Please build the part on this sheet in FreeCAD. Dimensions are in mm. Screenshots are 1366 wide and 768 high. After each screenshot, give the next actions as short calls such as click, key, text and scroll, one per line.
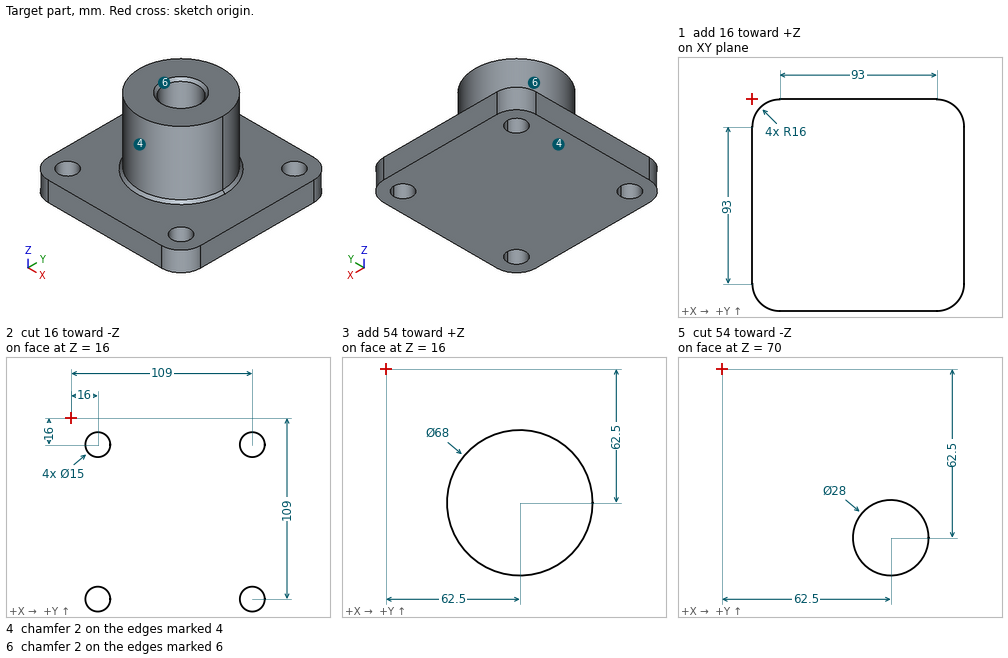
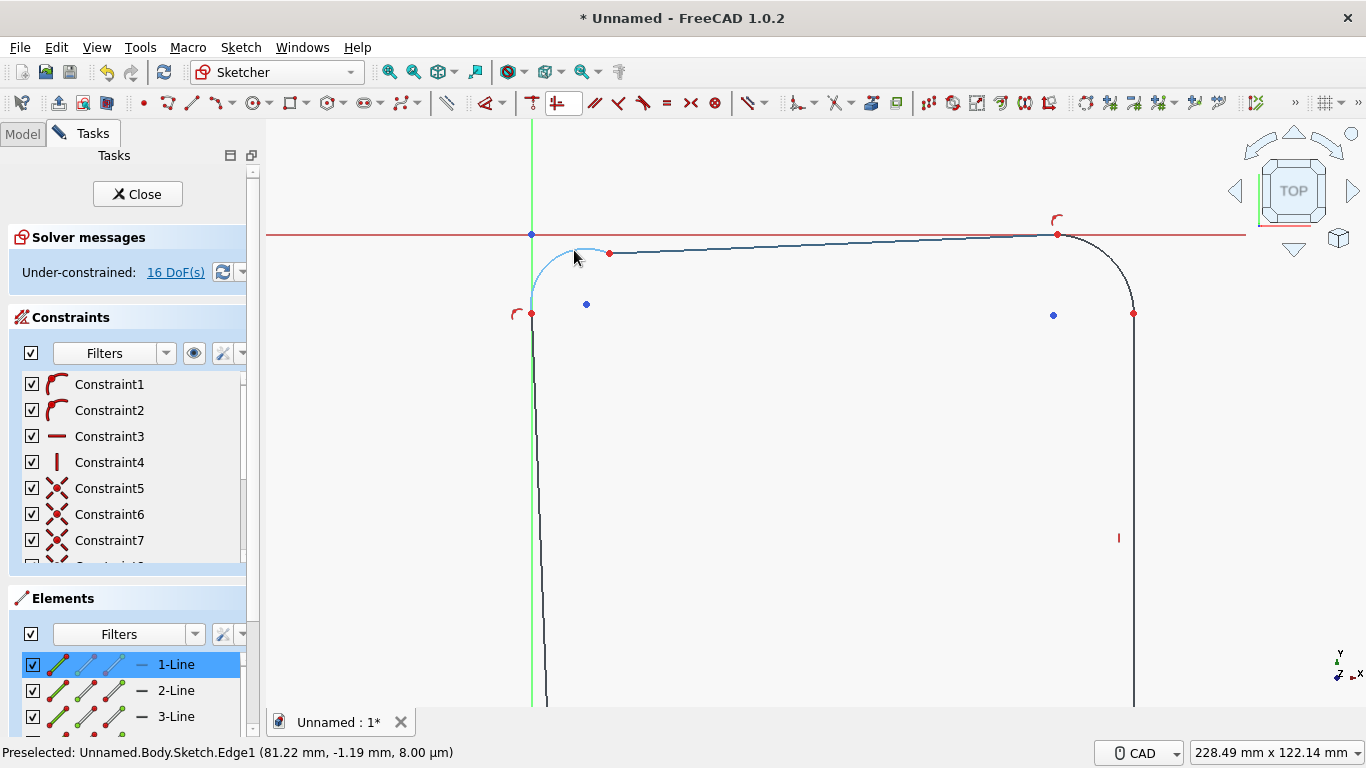
click(574, 250)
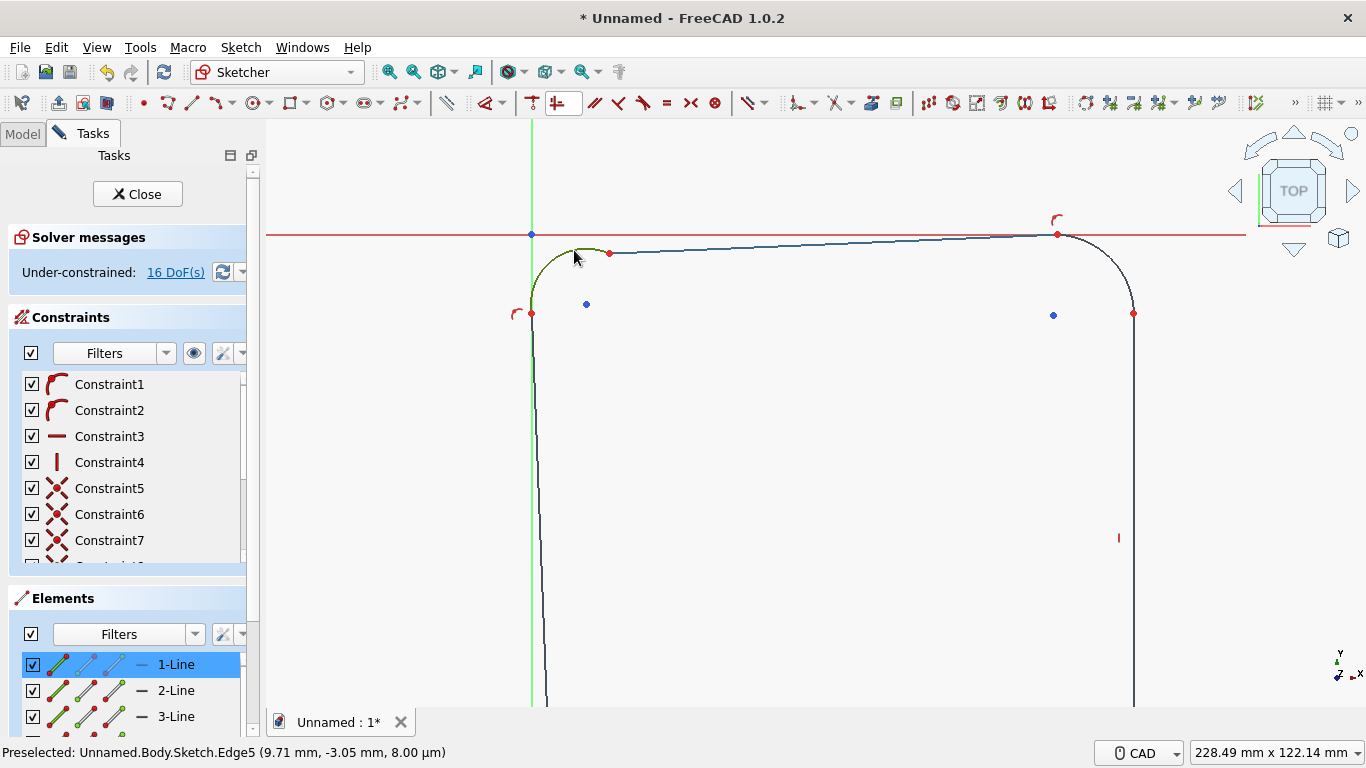
key(t)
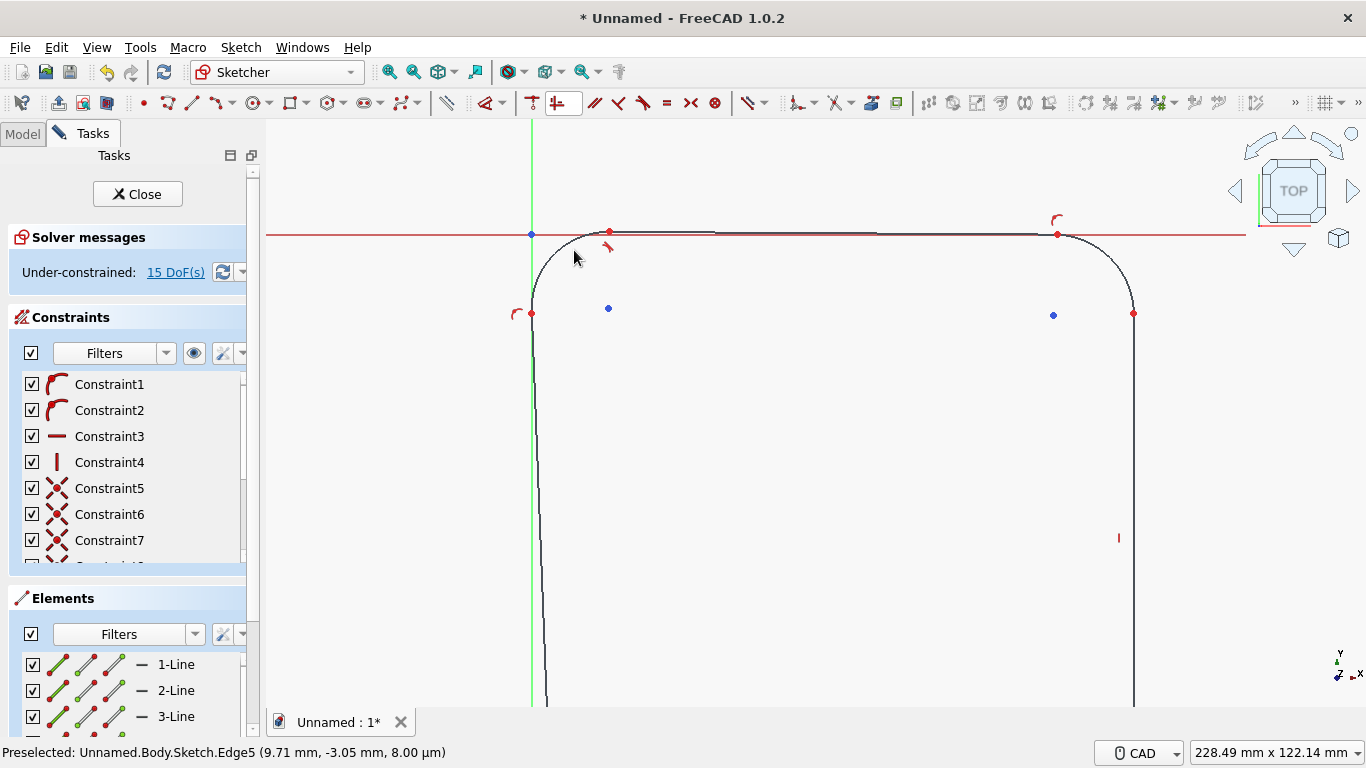
click(923, 234)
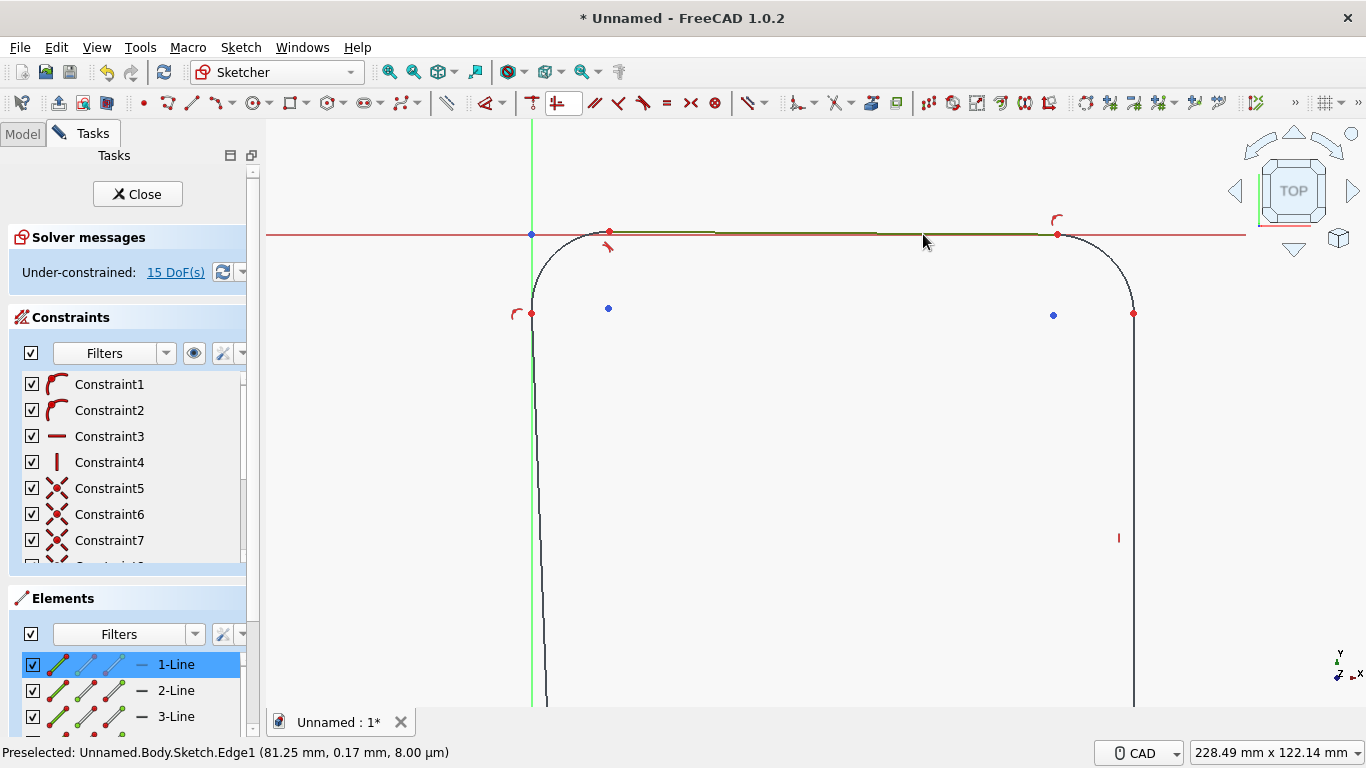
click(1125, 279)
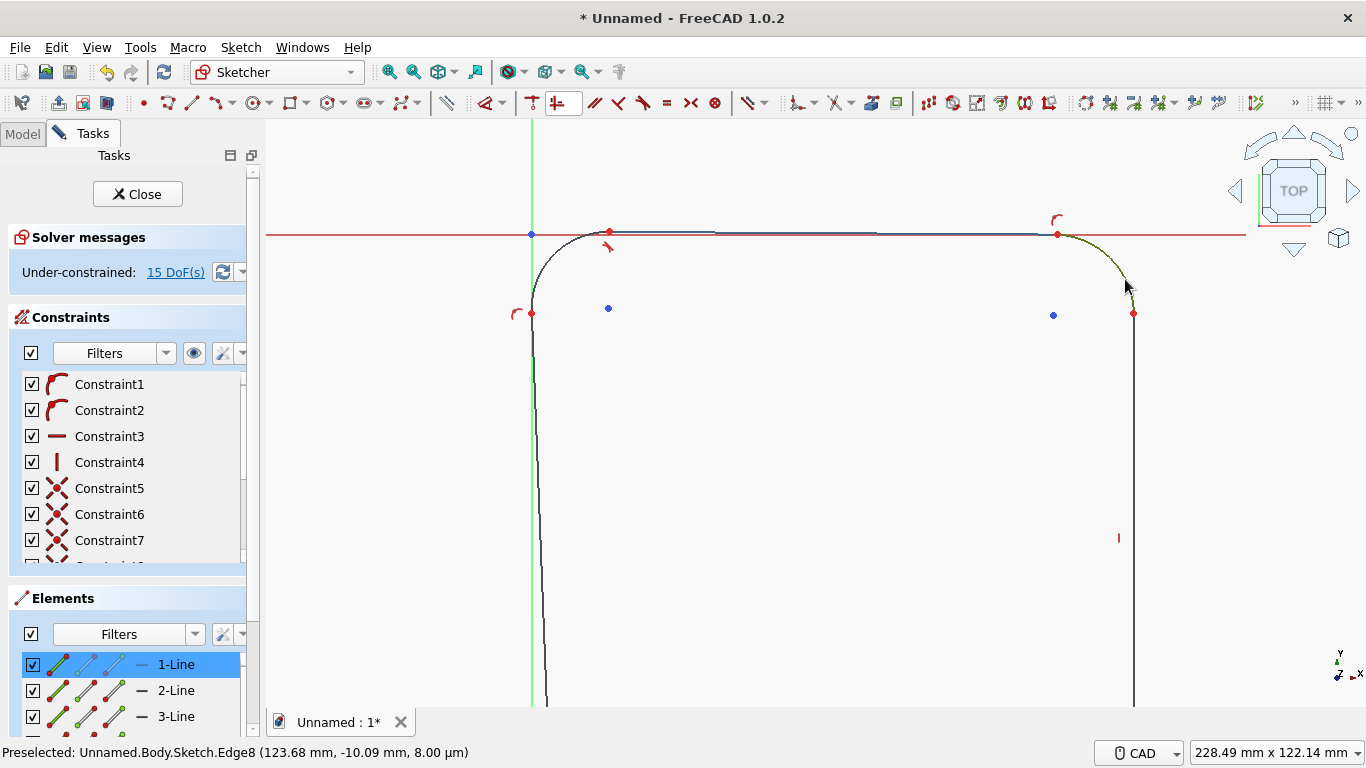
key(t)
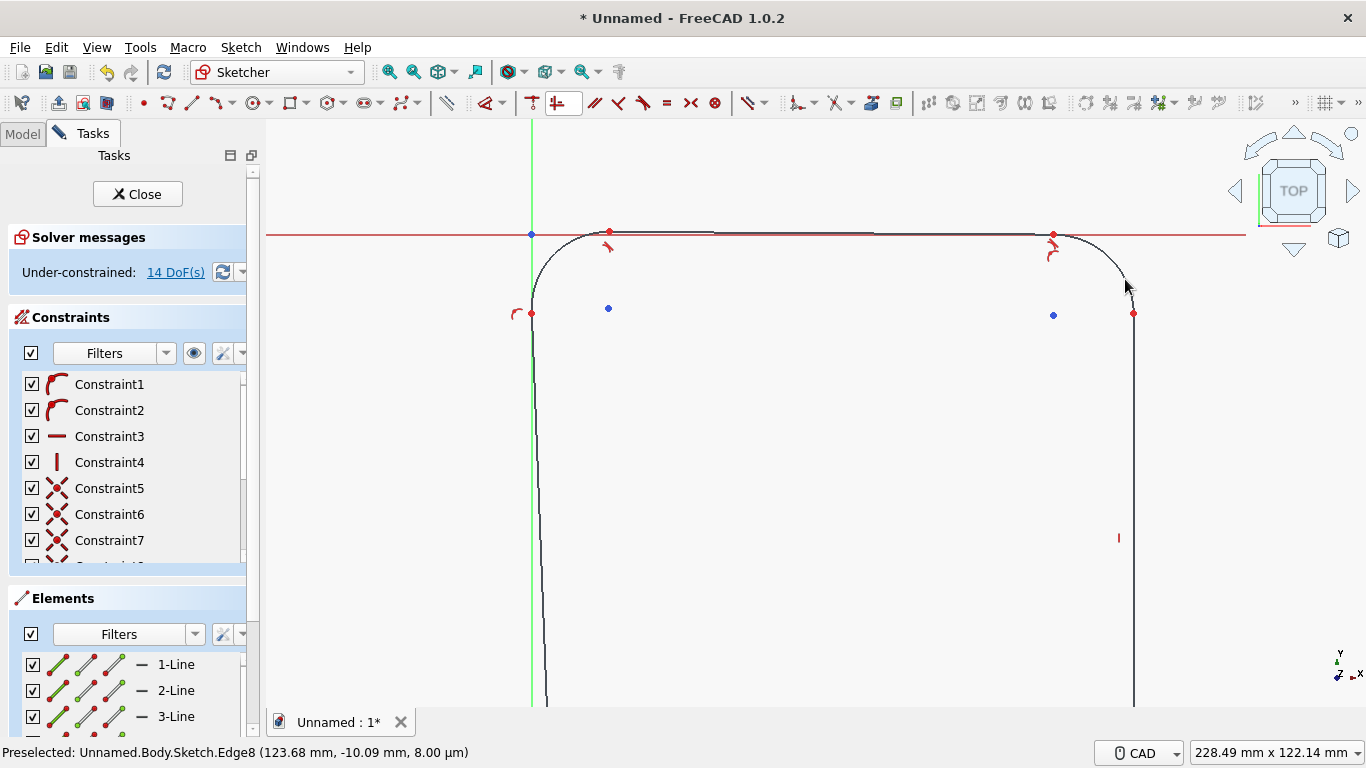
click(544, 628)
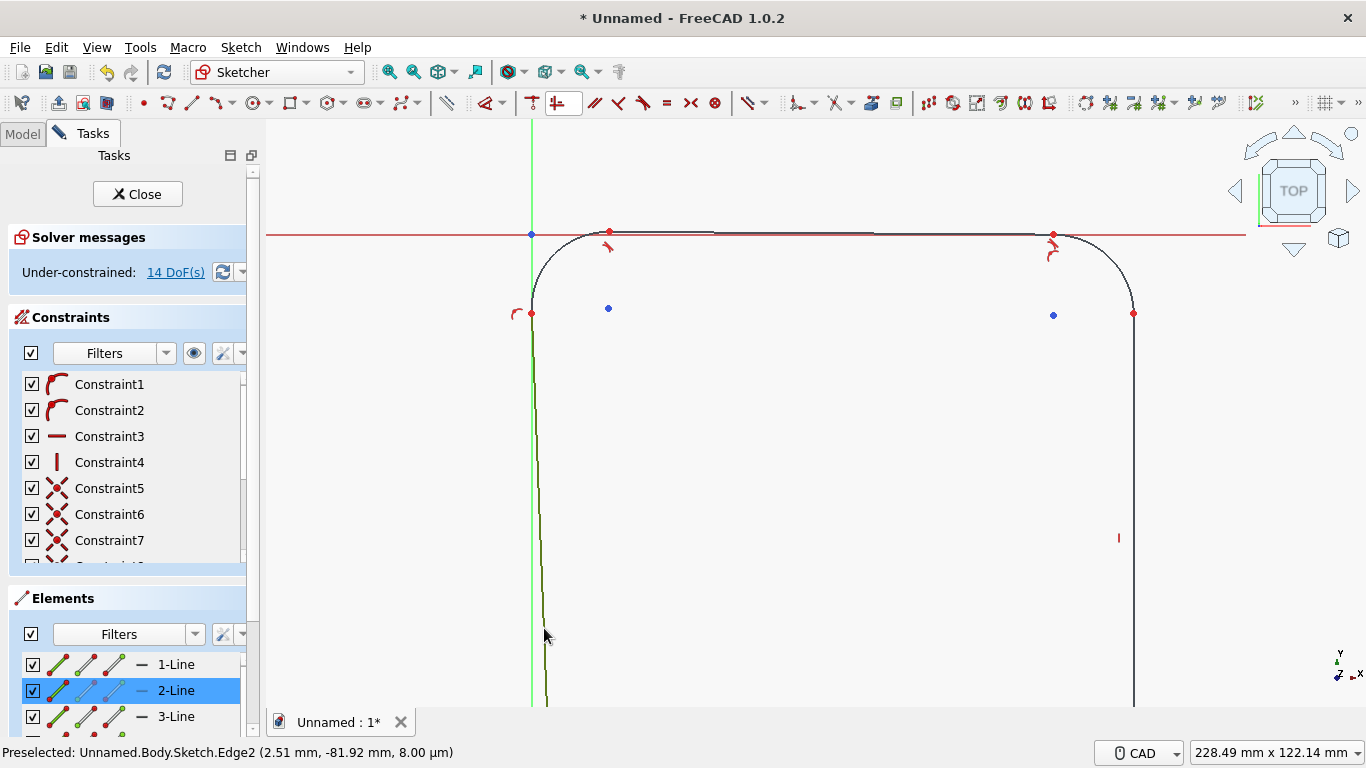
click(553, 256)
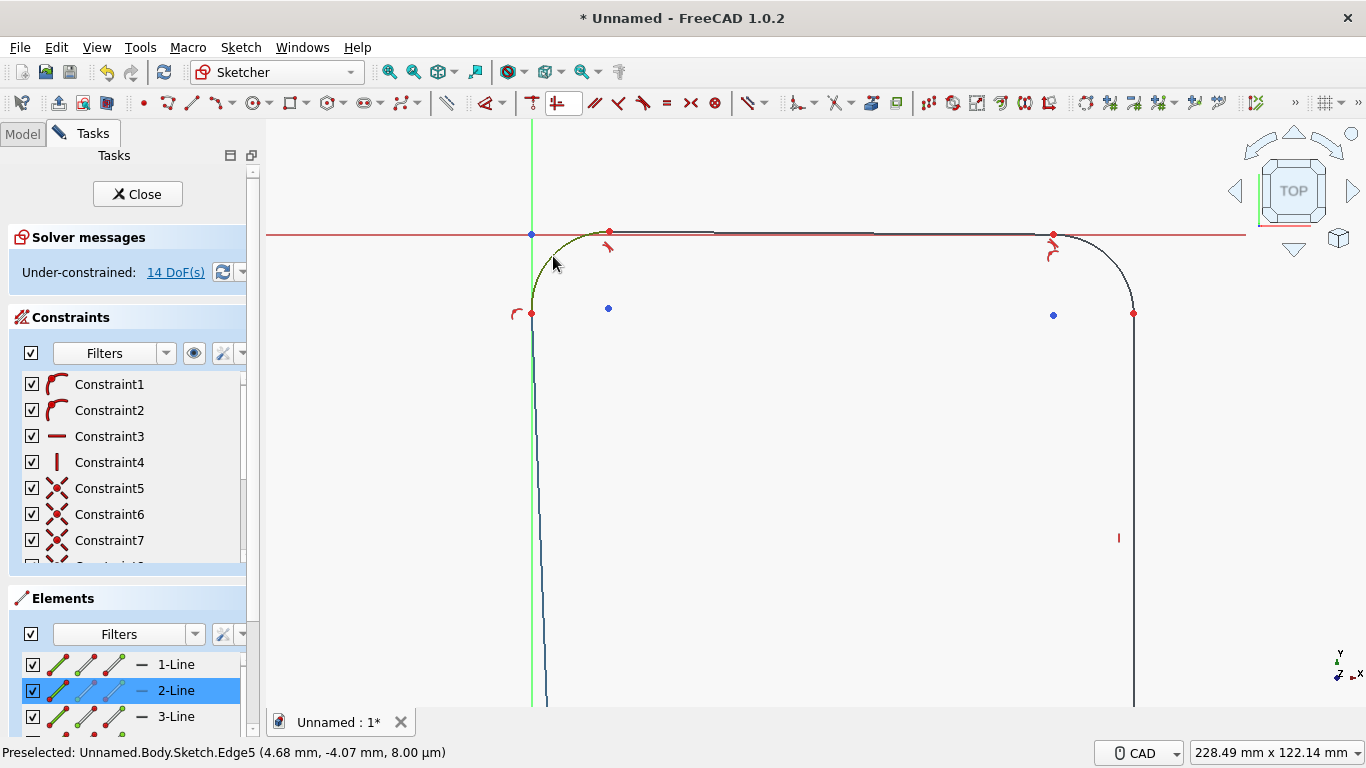
key(t)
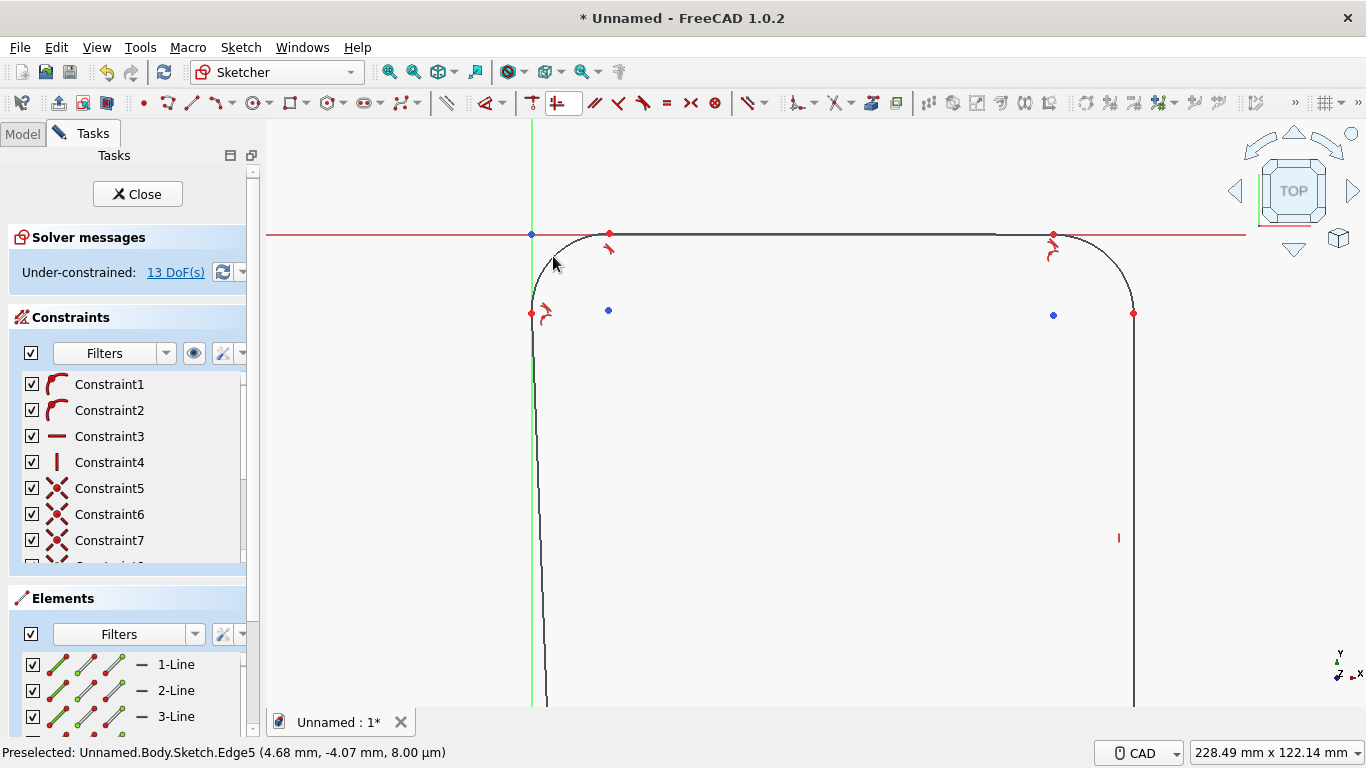
click(544, 628)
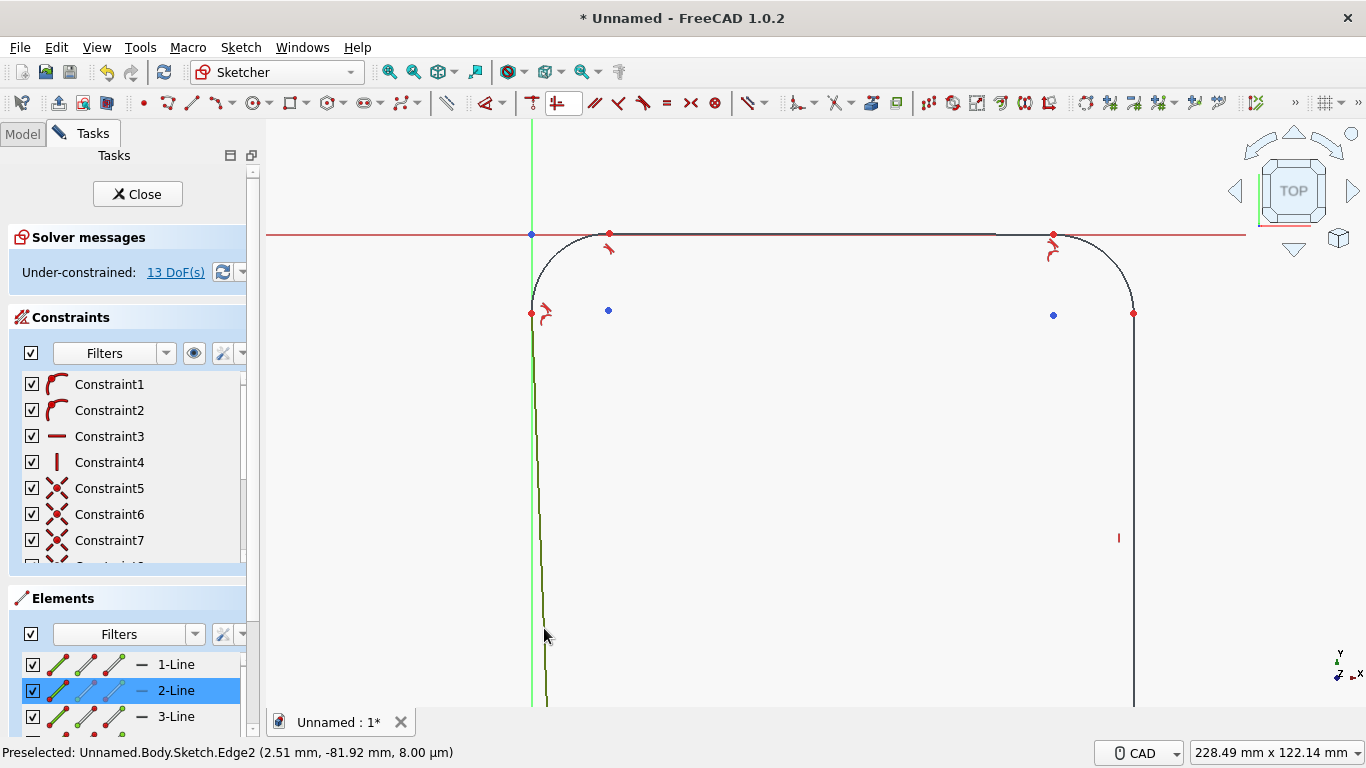
scroll(574, 164, down, 2)